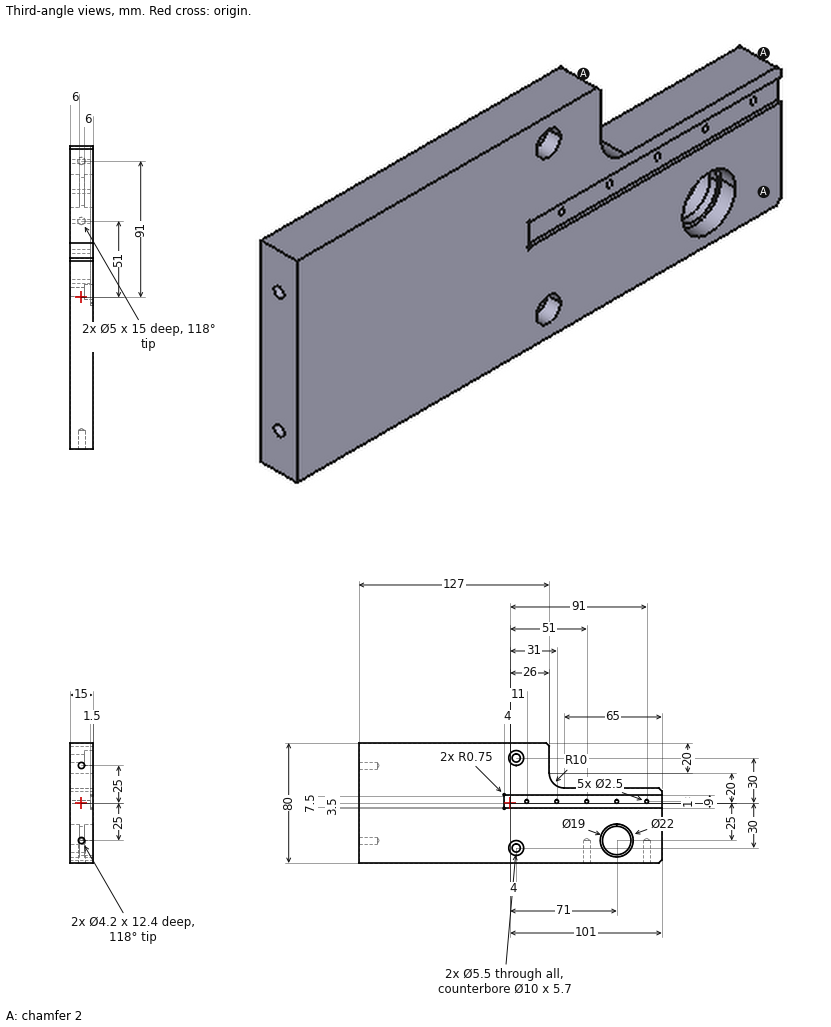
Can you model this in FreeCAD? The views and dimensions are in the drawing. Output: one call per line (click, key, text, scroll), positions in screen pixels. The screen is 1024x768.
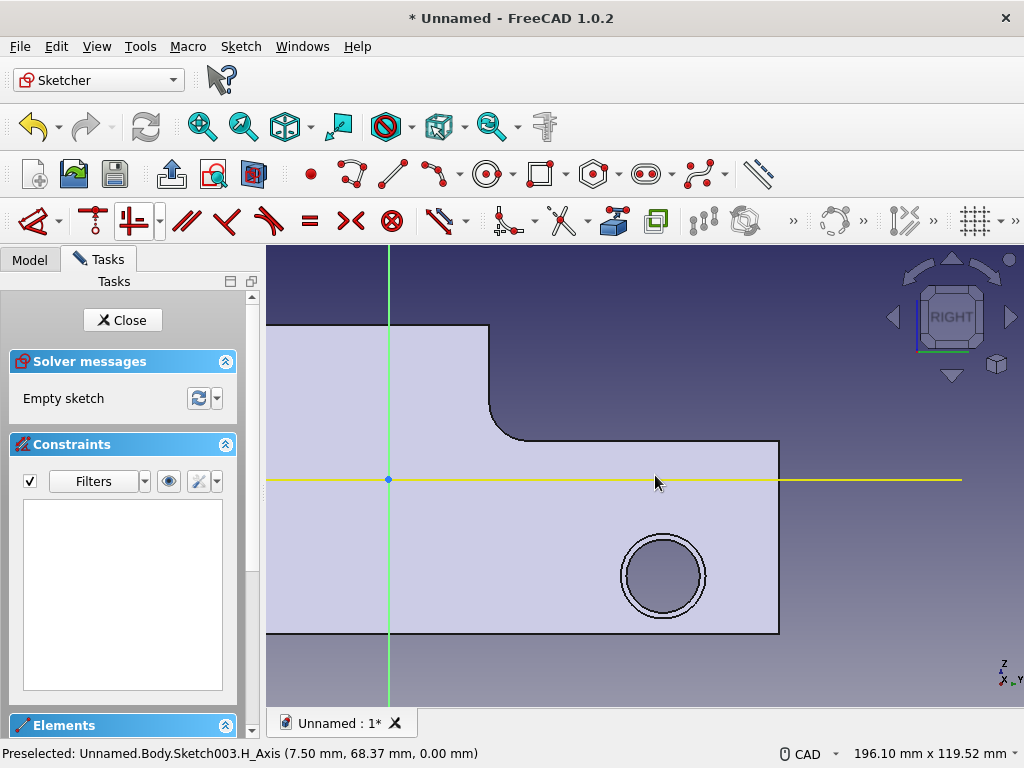
click(393, 174)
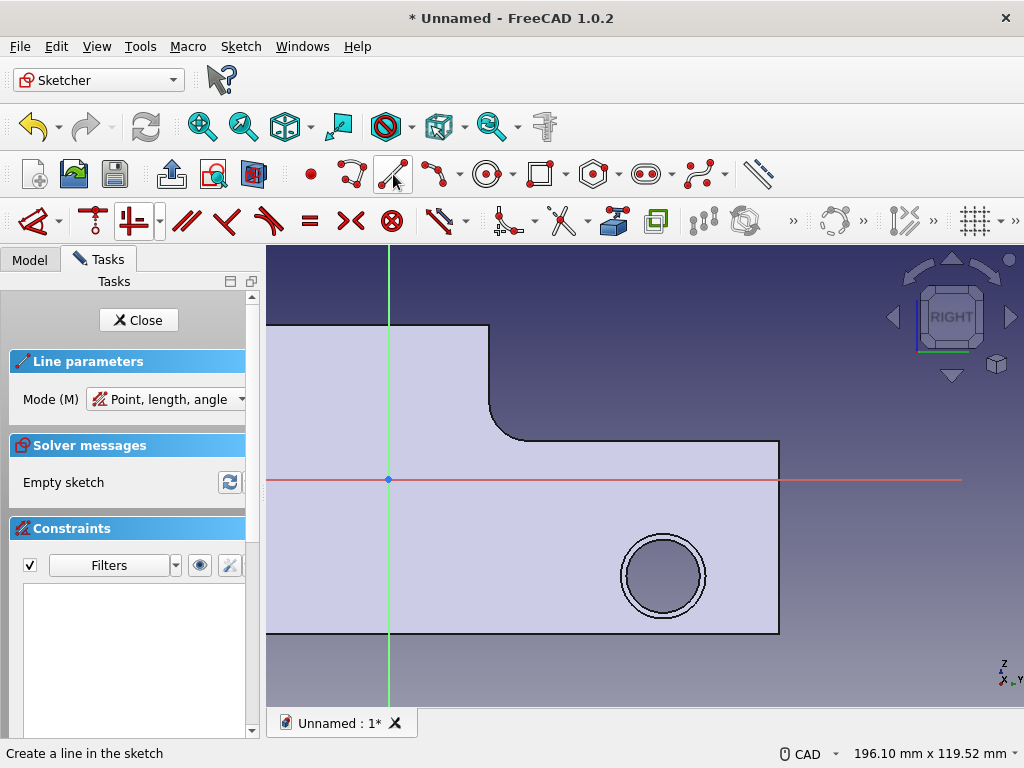
click(373, 461)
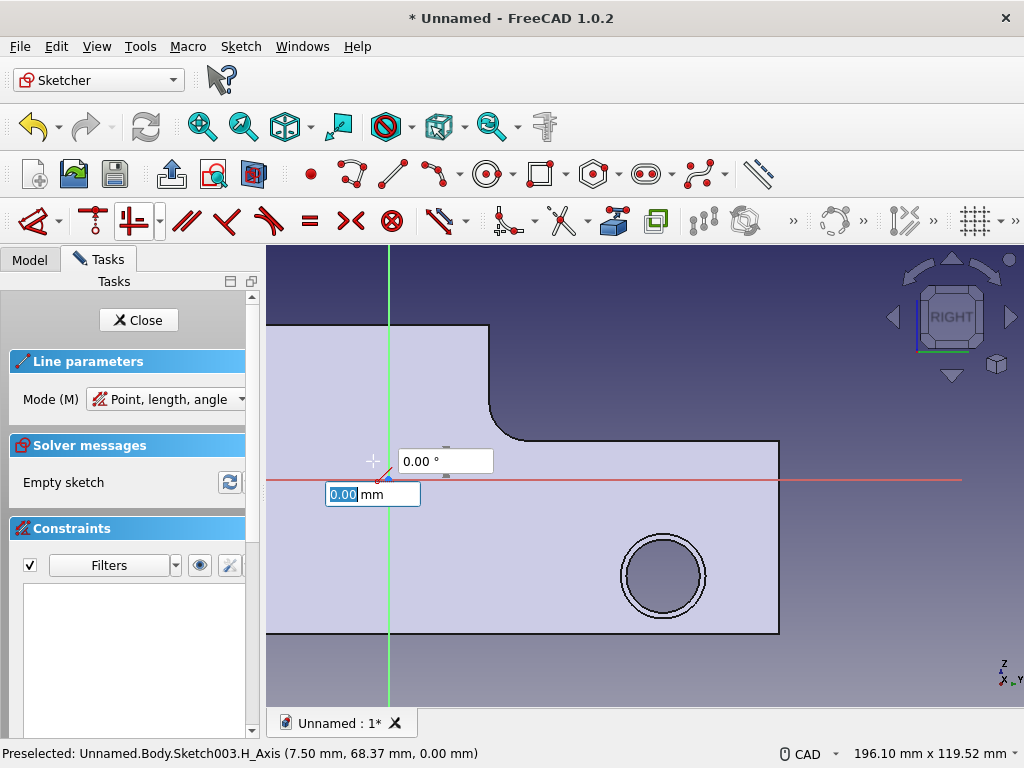
scroll(373, 490, up, 3)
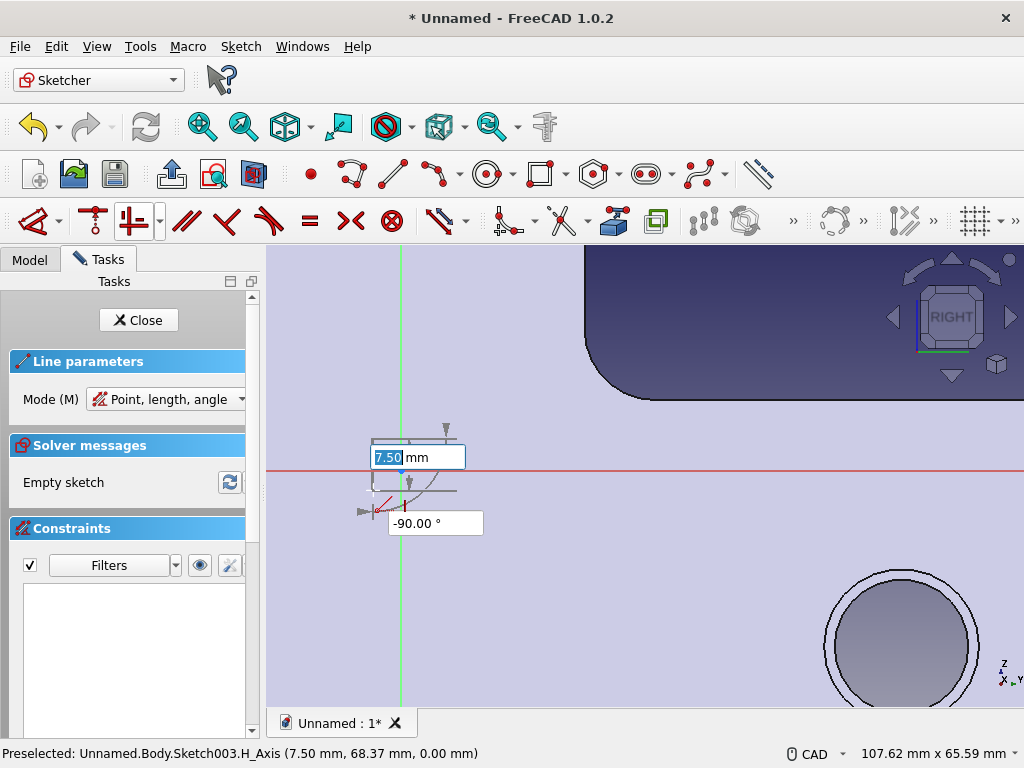
click(373, 490)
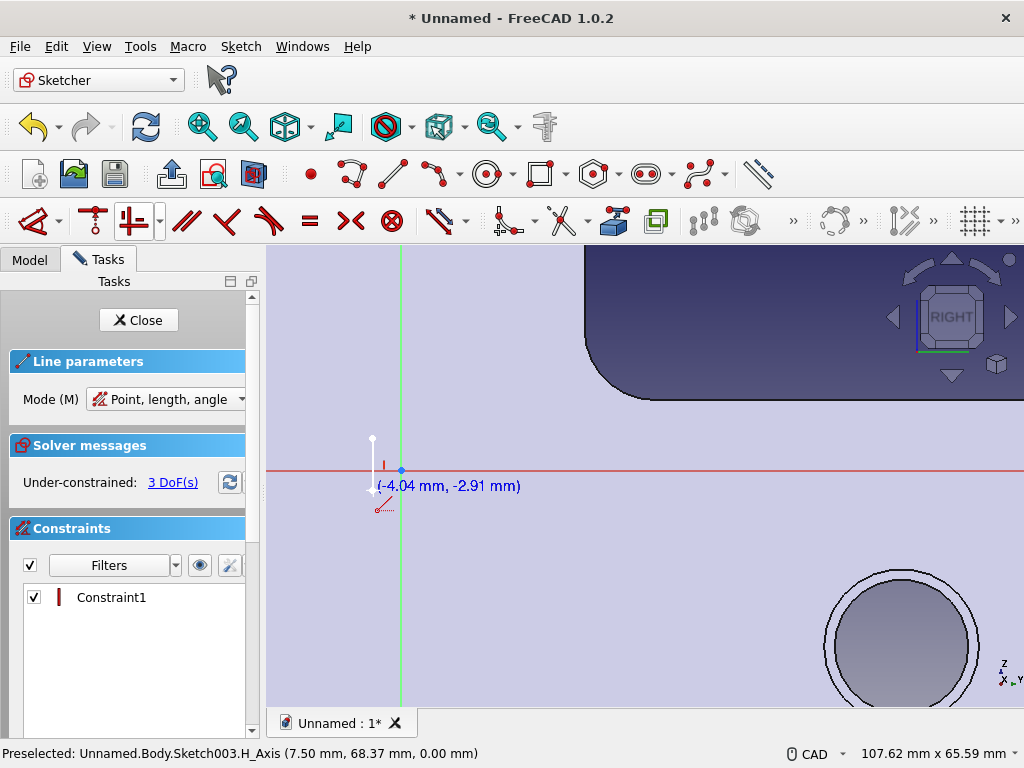
click(352, 174)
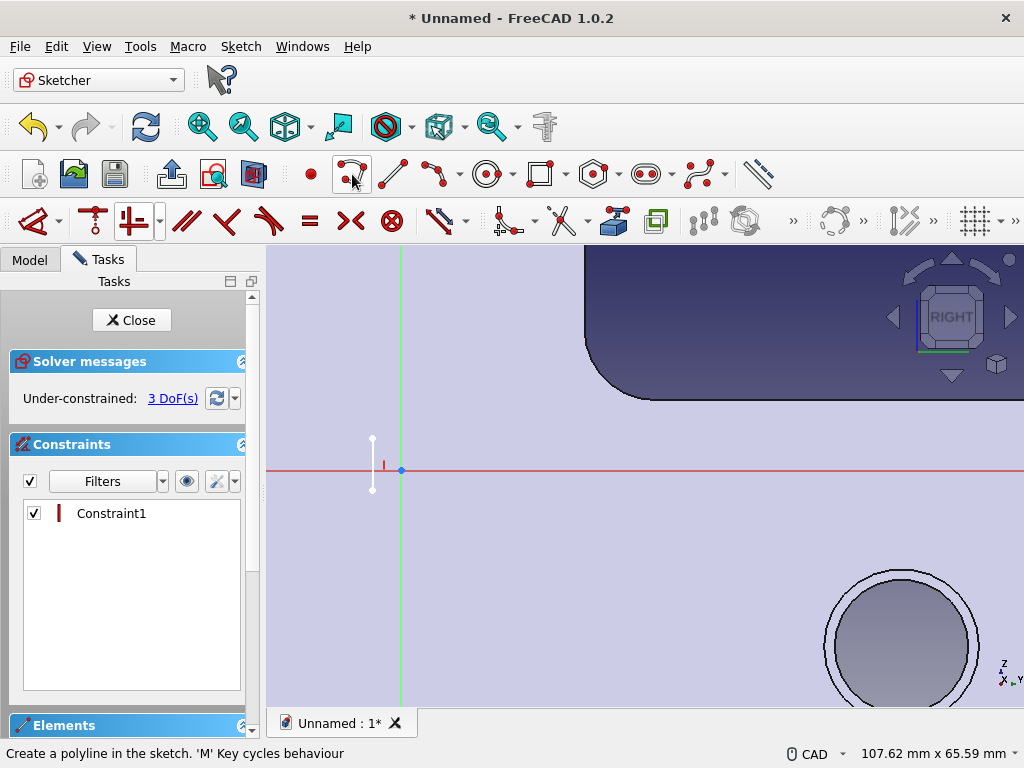
scroll(379, 495, up, 4)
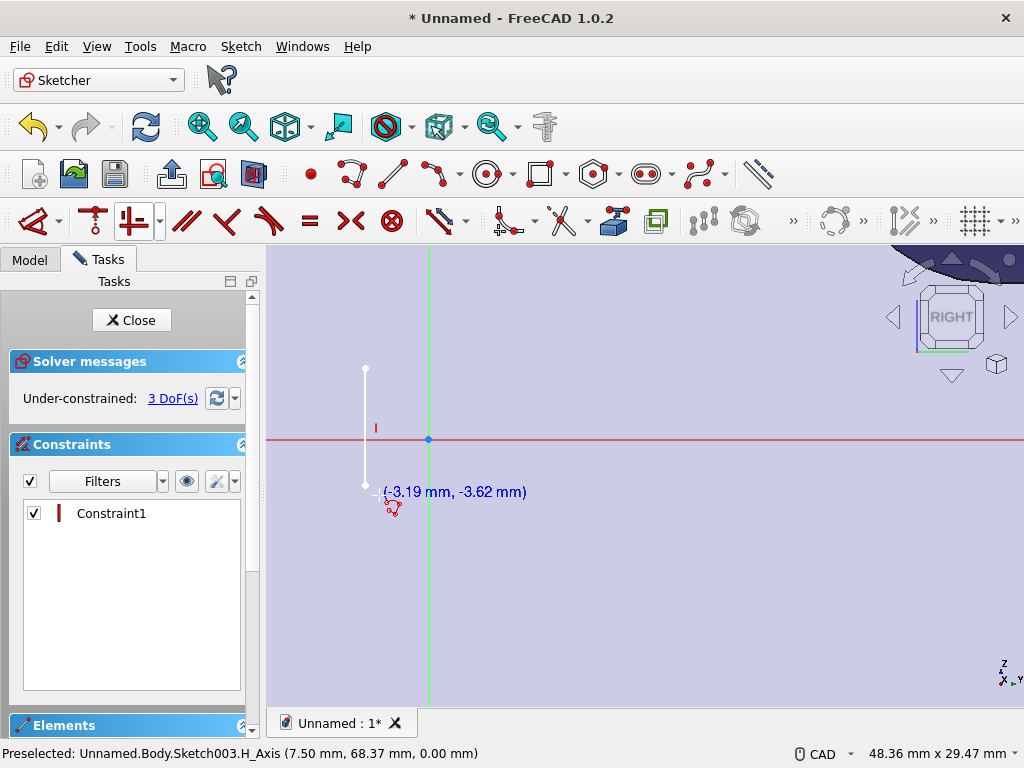
click(378, 495)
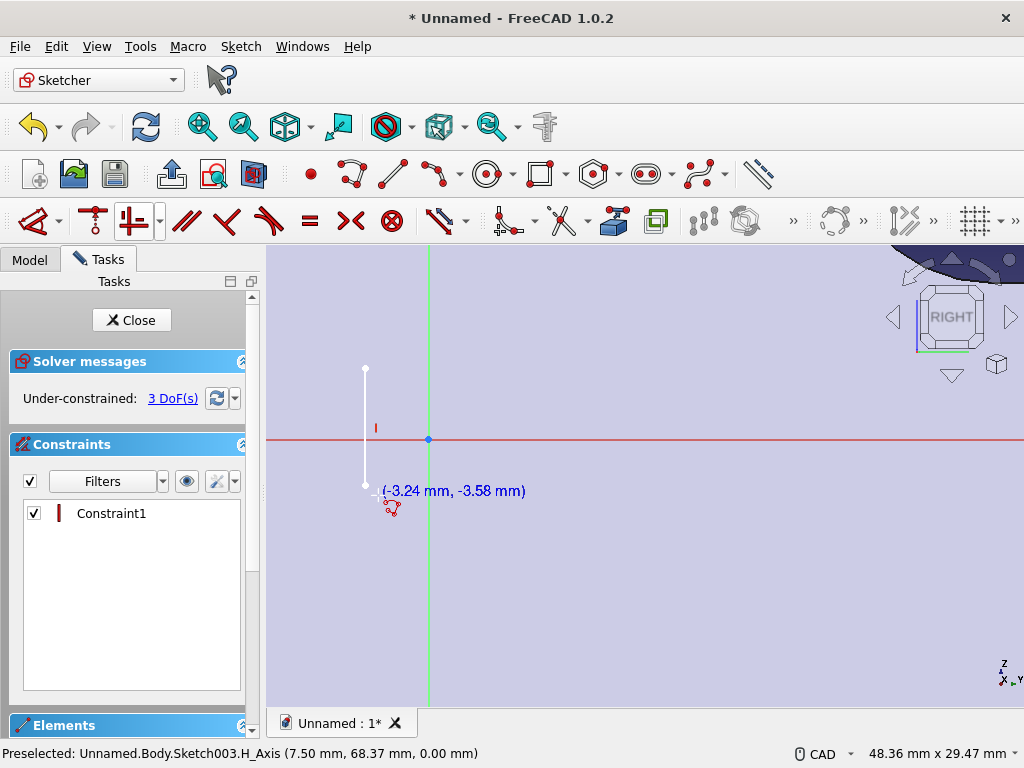
scroll(377, 493, down, 7)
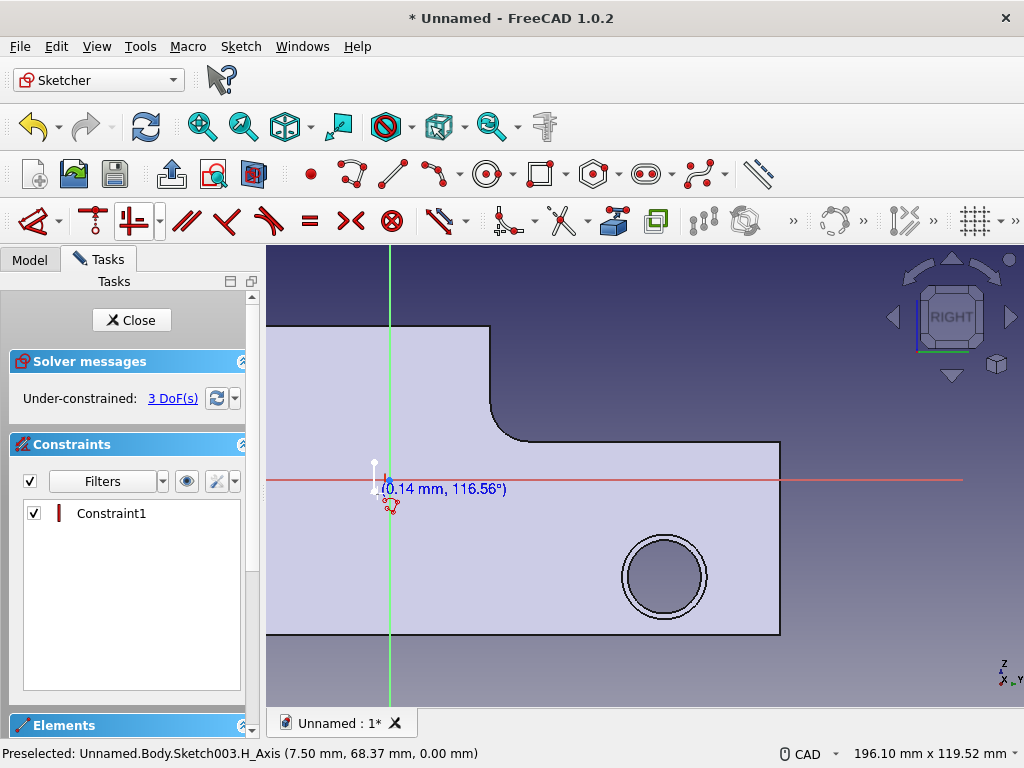
click(780, 494)
click(780, 459)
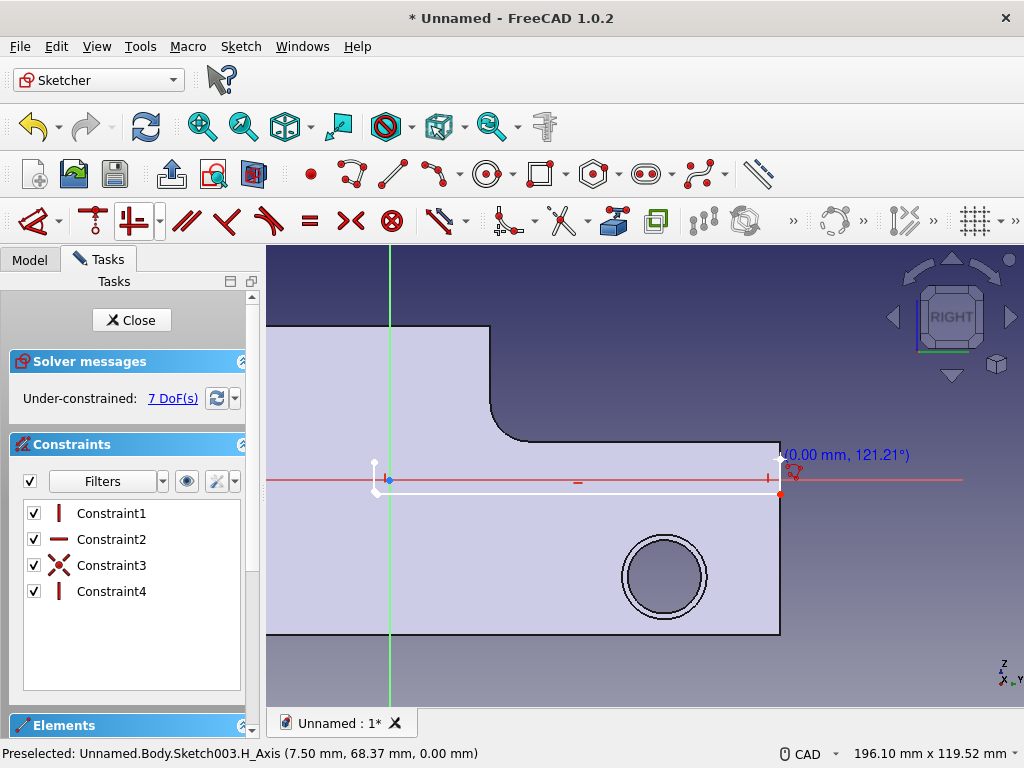
scroll(377, 459, up, 7)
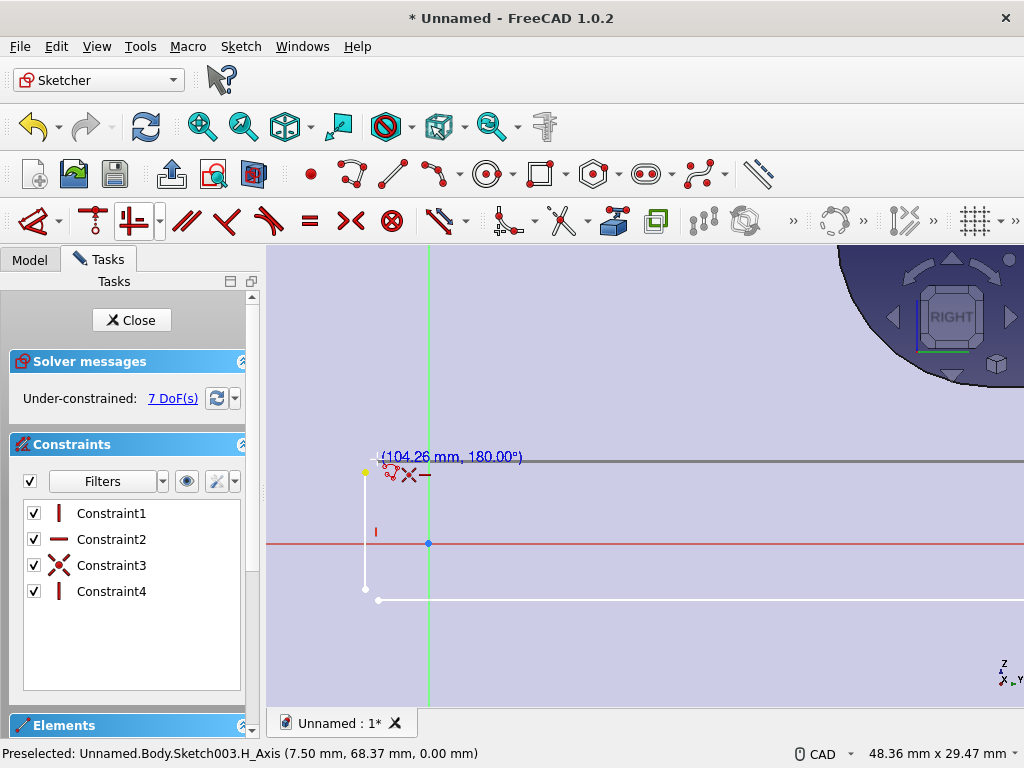
click(378, 458)
right_click(378, 458)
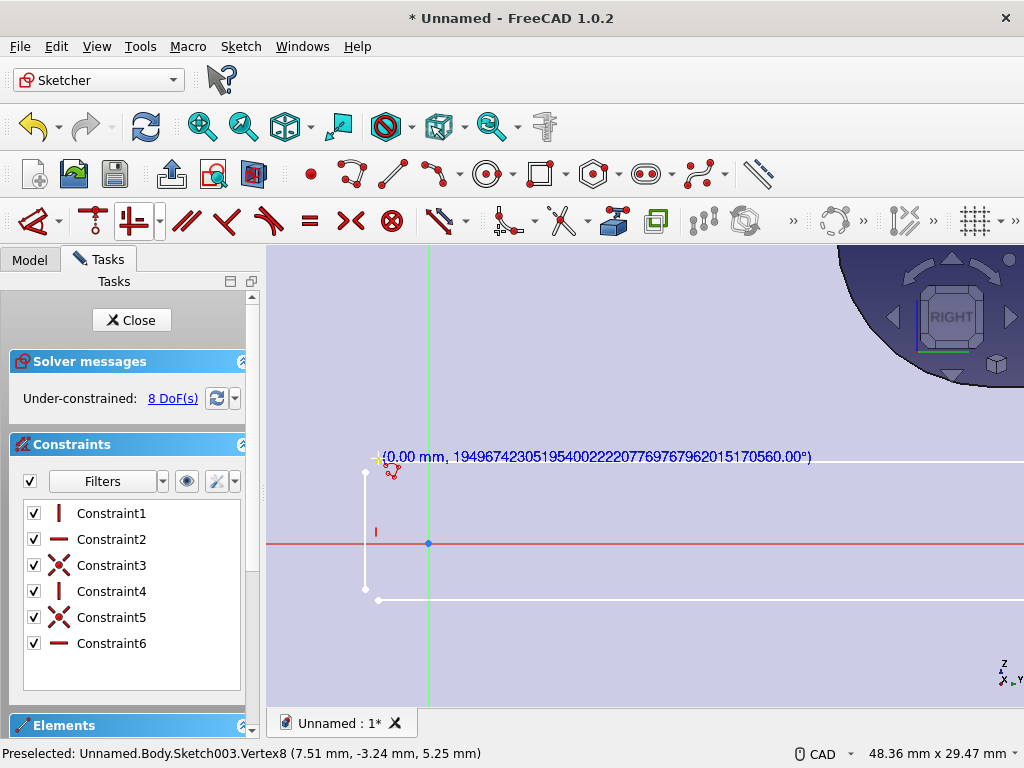
click(434, 174)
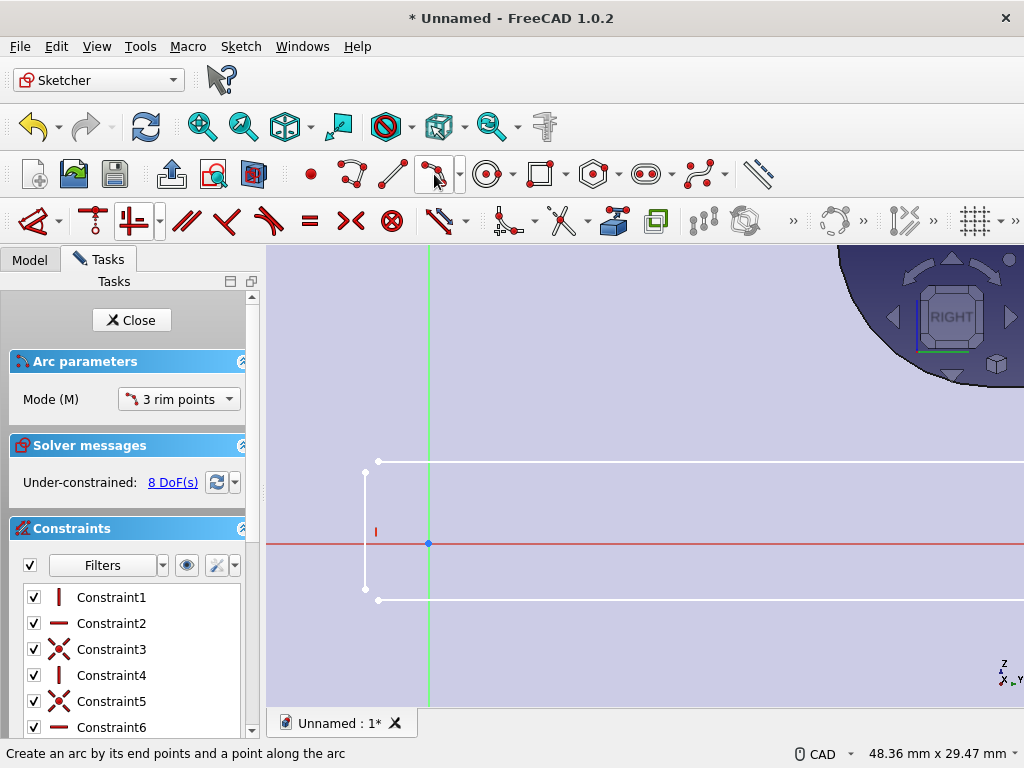
click(365, 590)
click(378, 600)
click(358, 607)